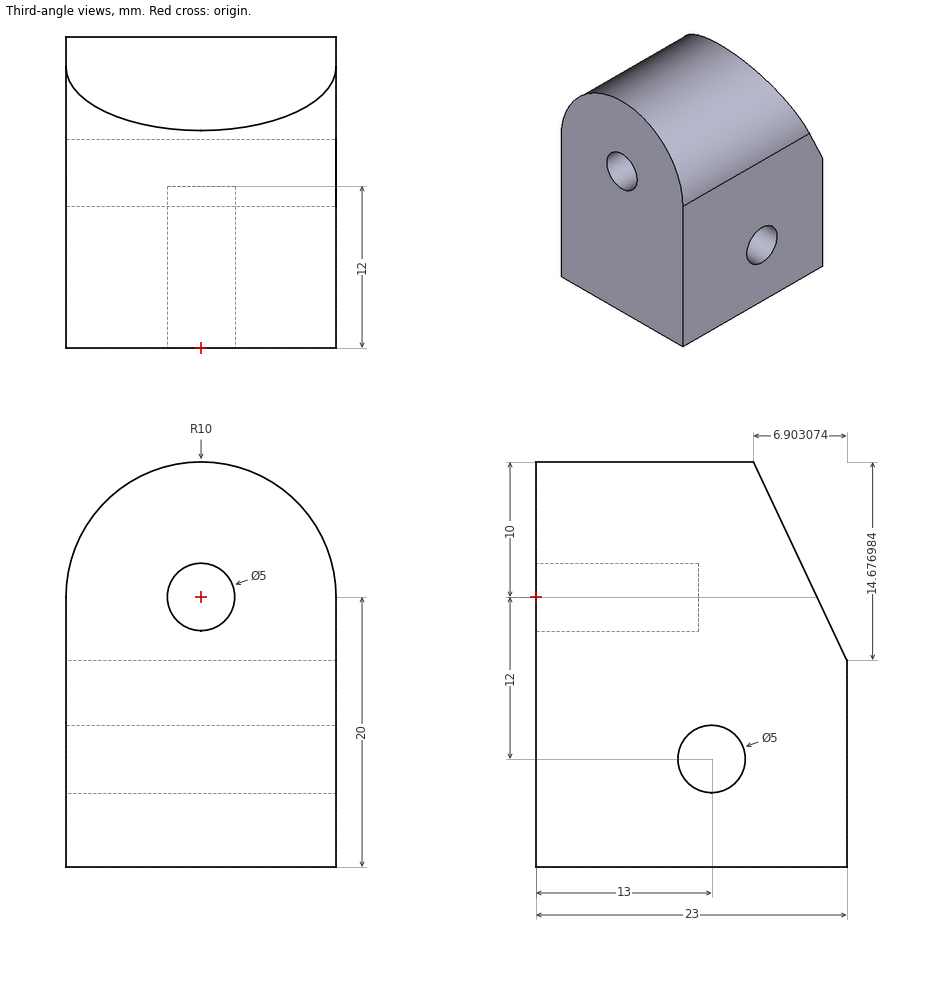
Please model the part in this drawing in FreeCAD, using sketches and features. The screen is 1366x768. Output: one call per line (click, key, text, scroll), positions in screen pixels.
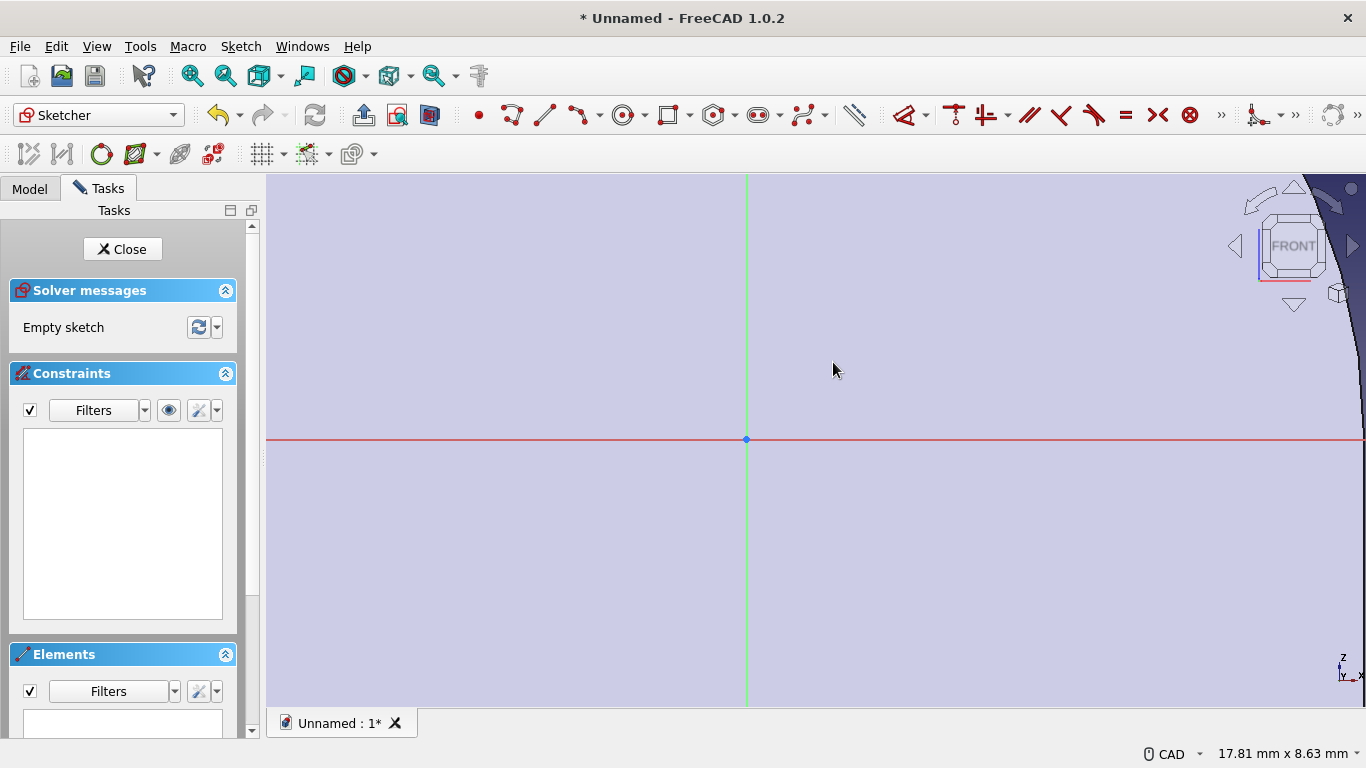
key(g)
key(c)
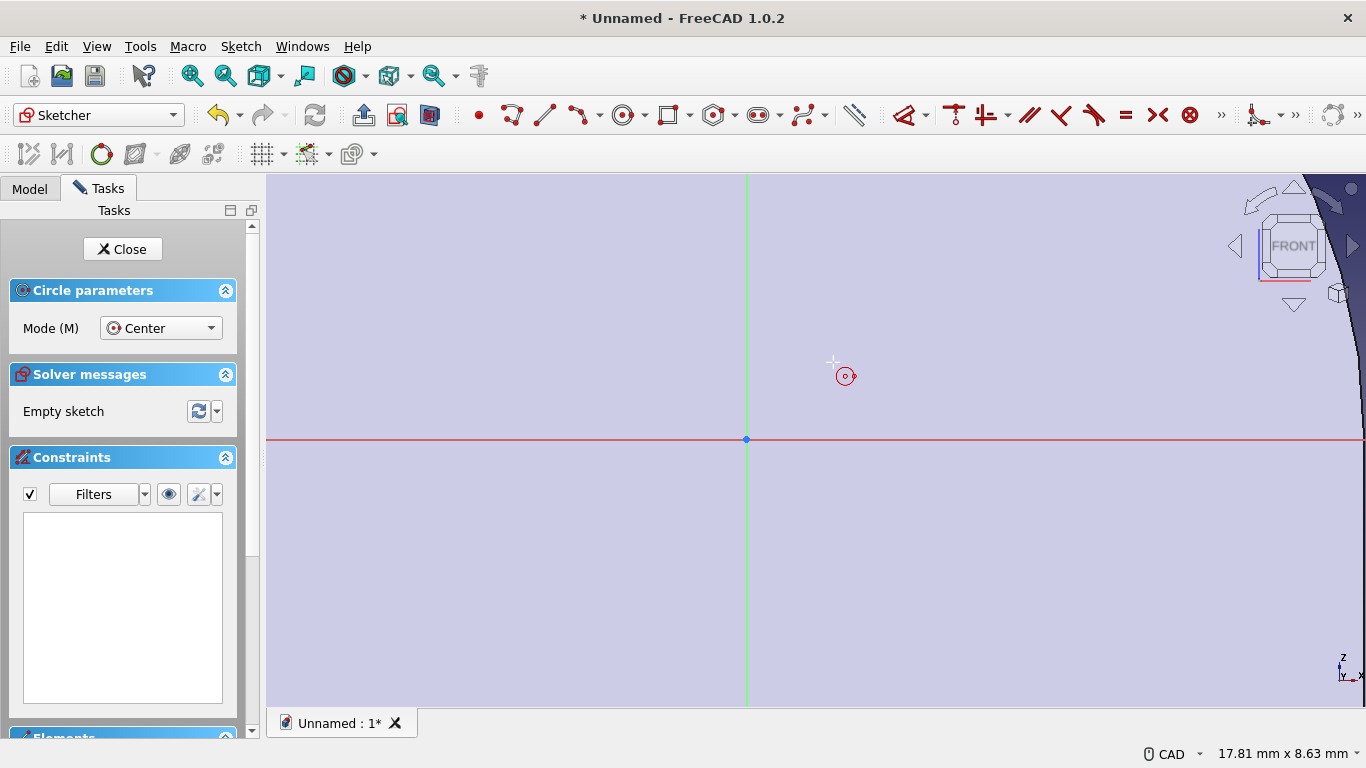
click(747, 440)
click(856, 331)
key(Escape)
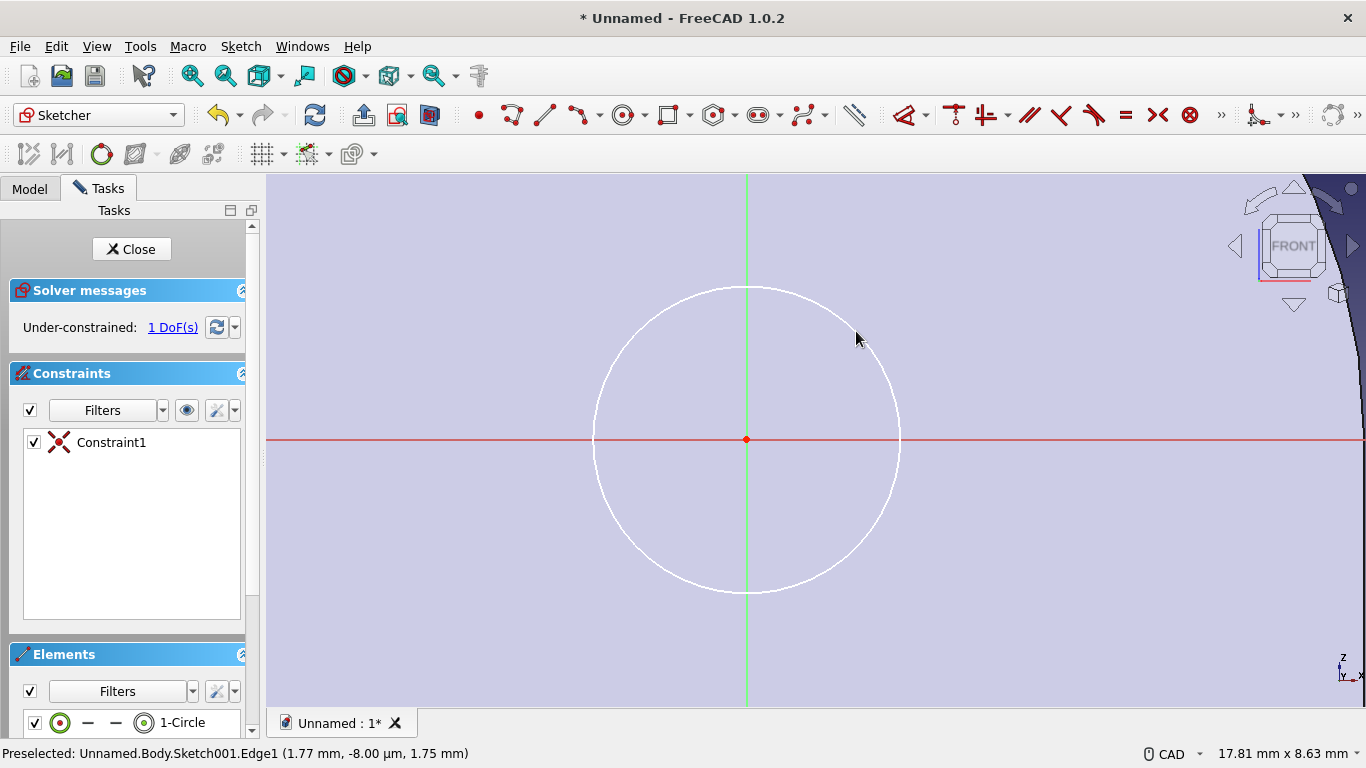
click(904, 116)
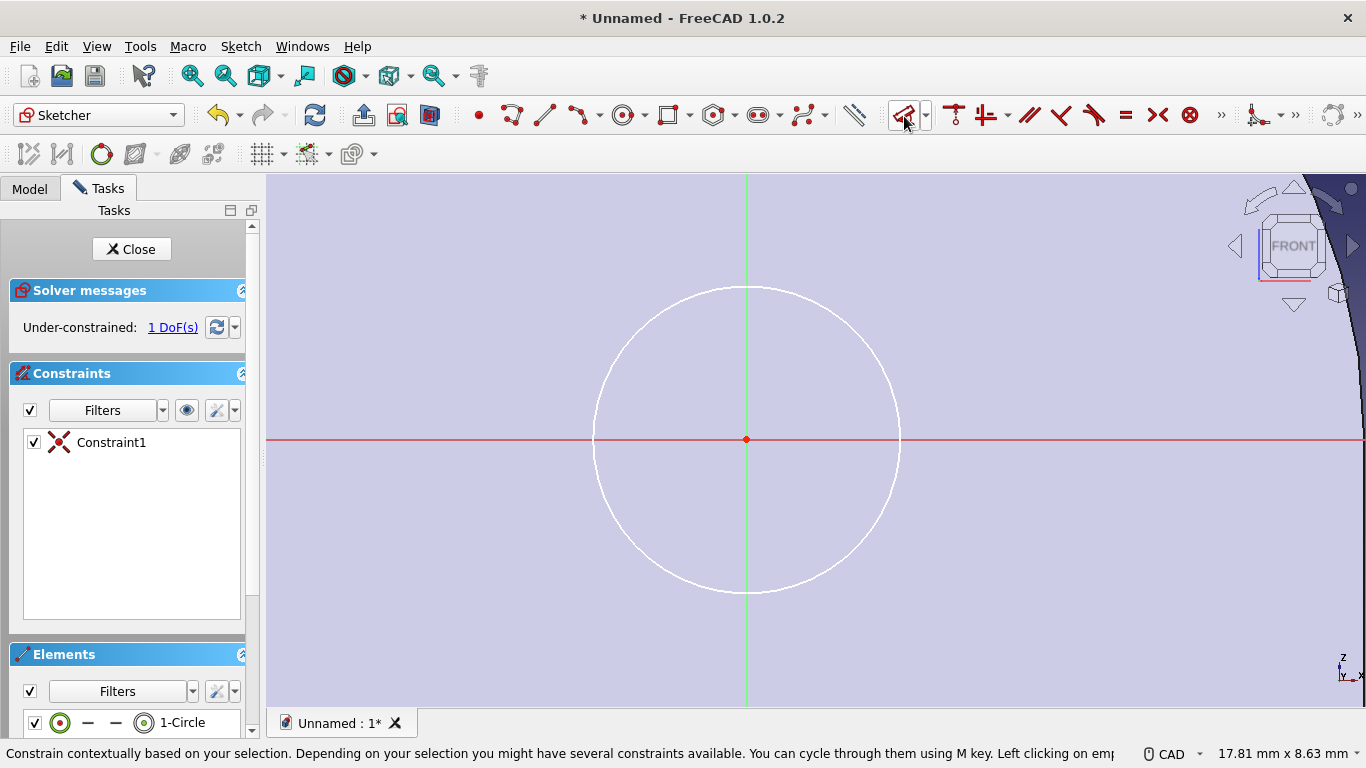
click(855, 331)
click(878, 308)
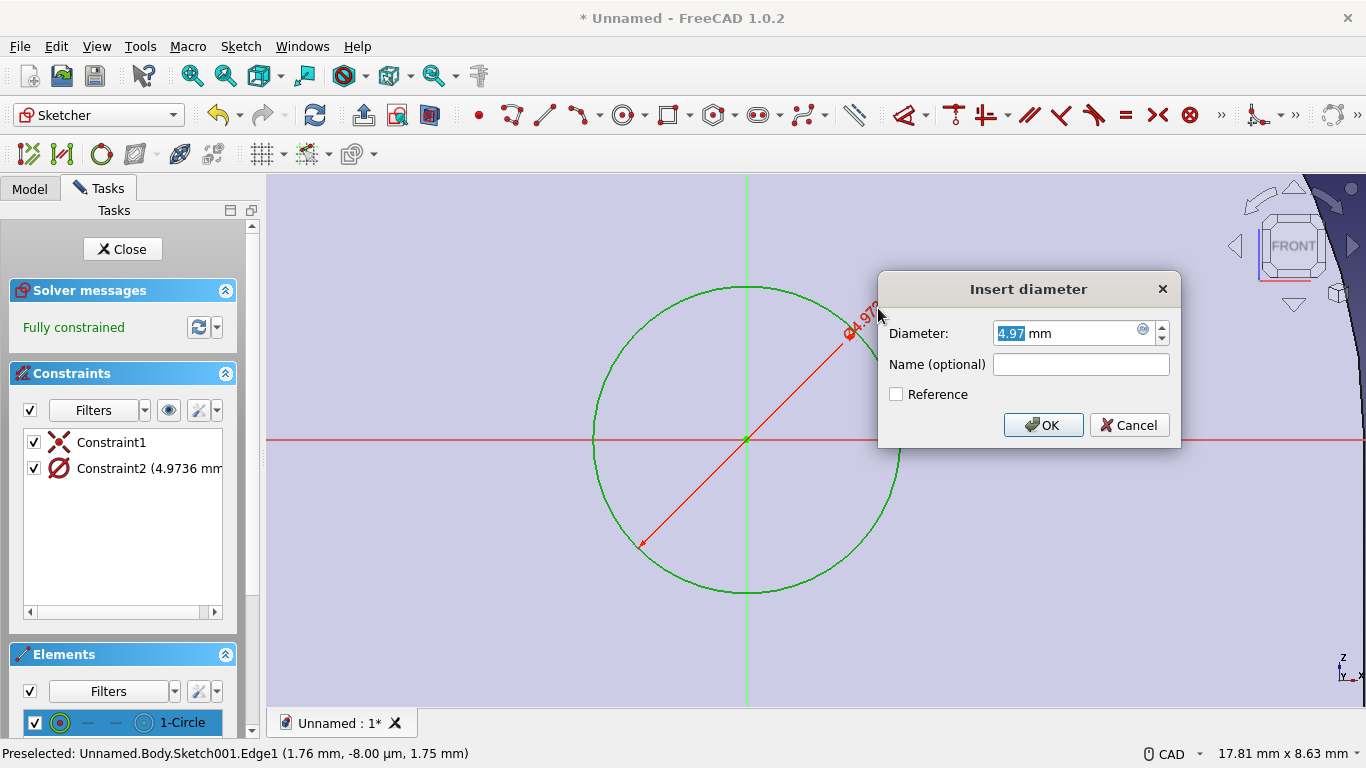
text(5)
key(Return)
key(Escape)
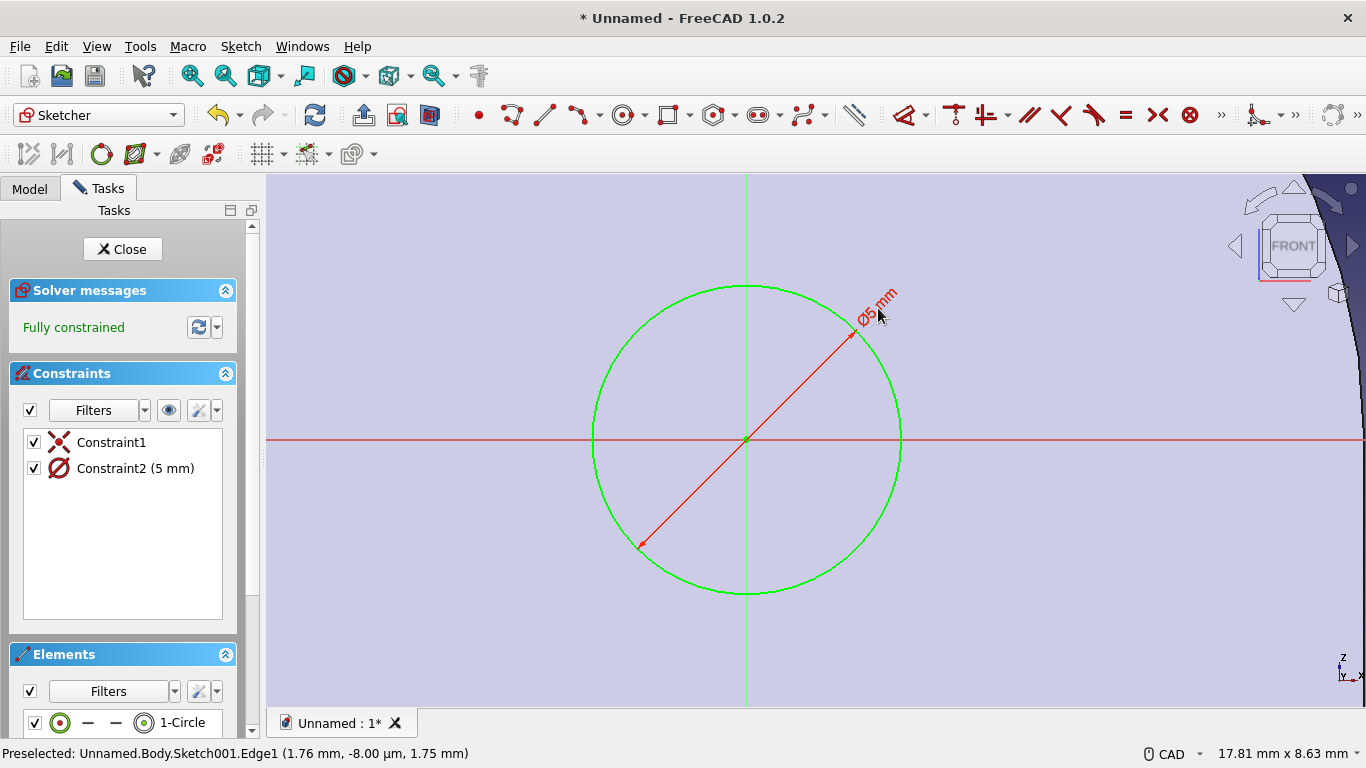
click(123, 249)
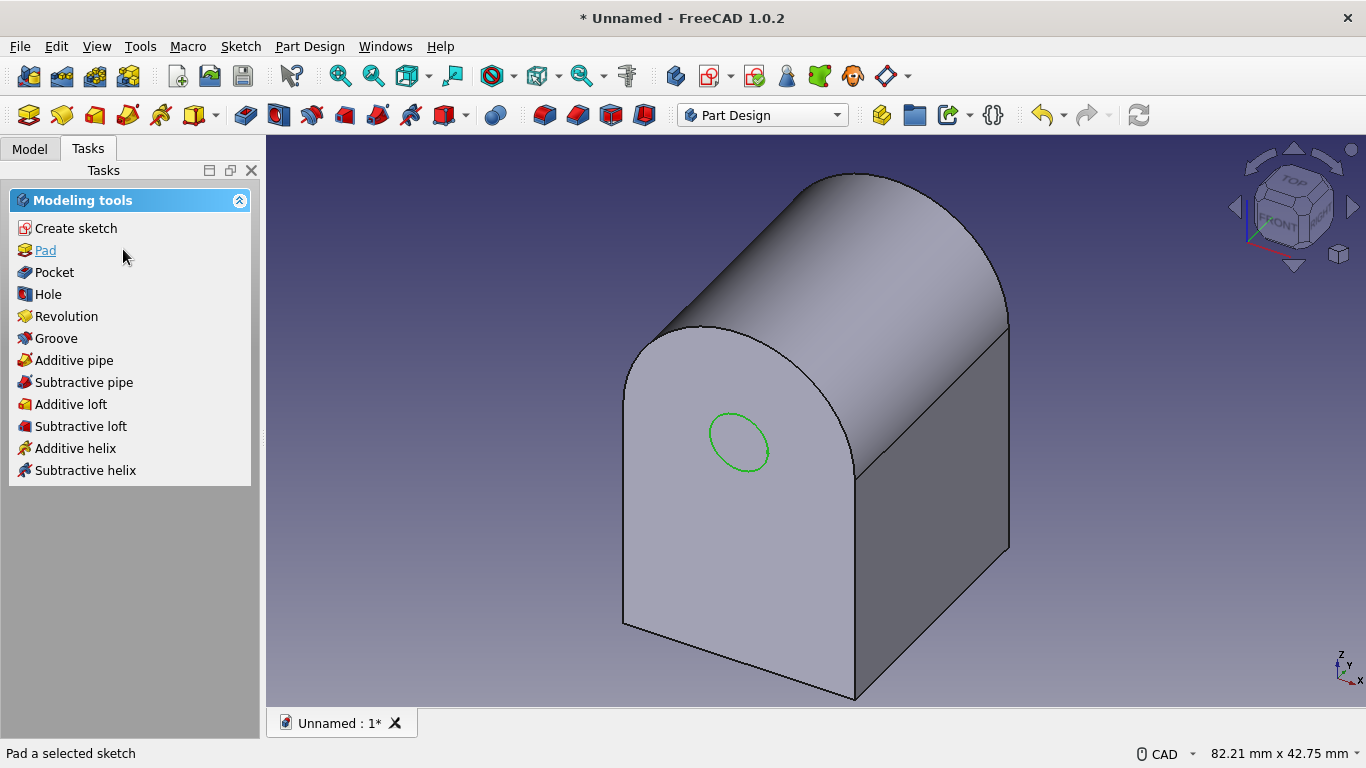
click(246, 116)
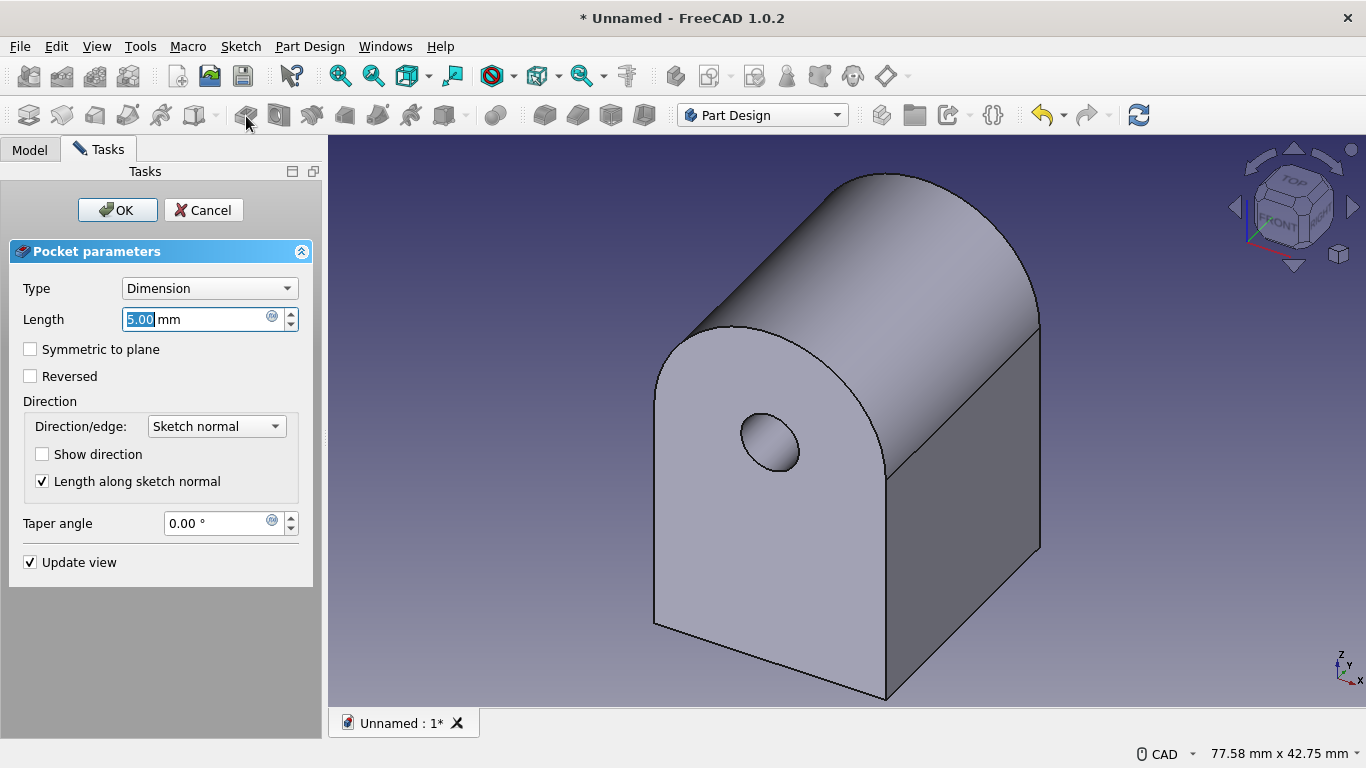
text(12)
key(Tab)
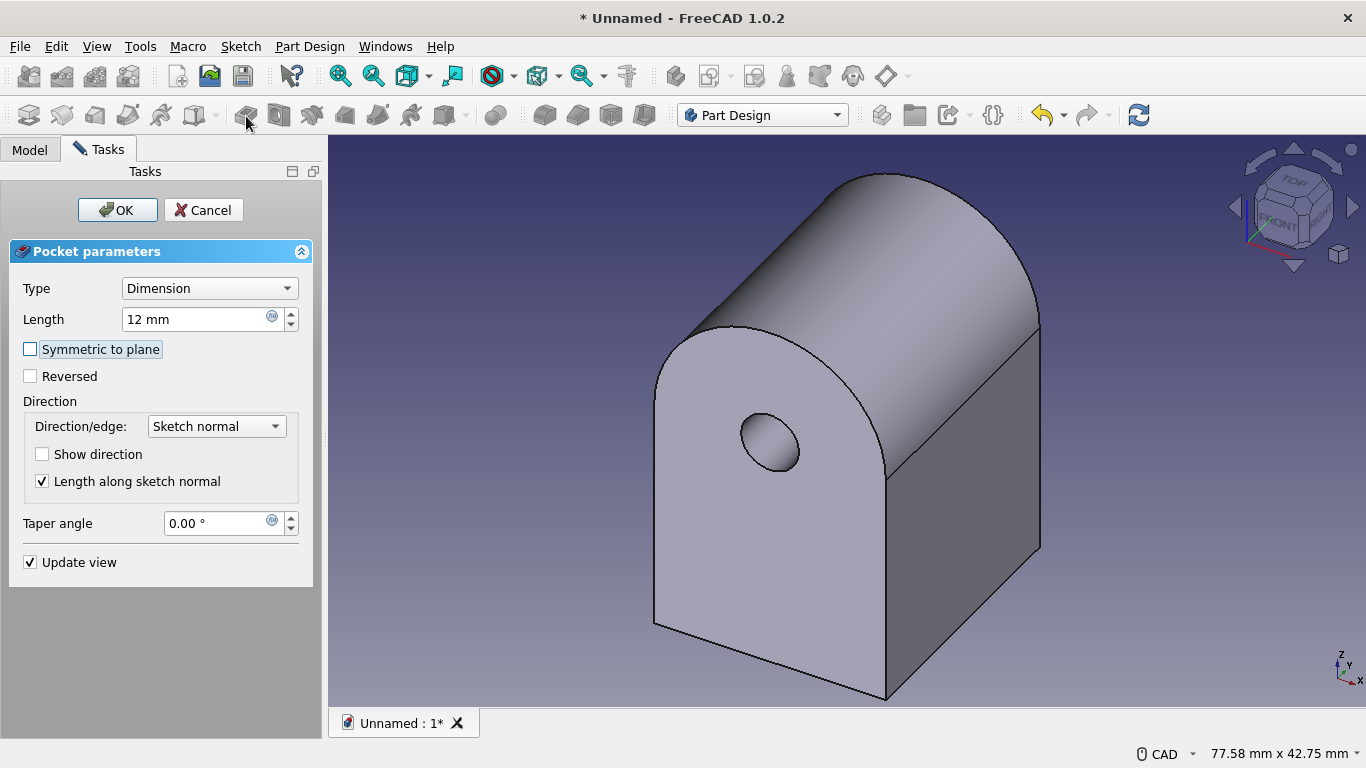
click(118, 210)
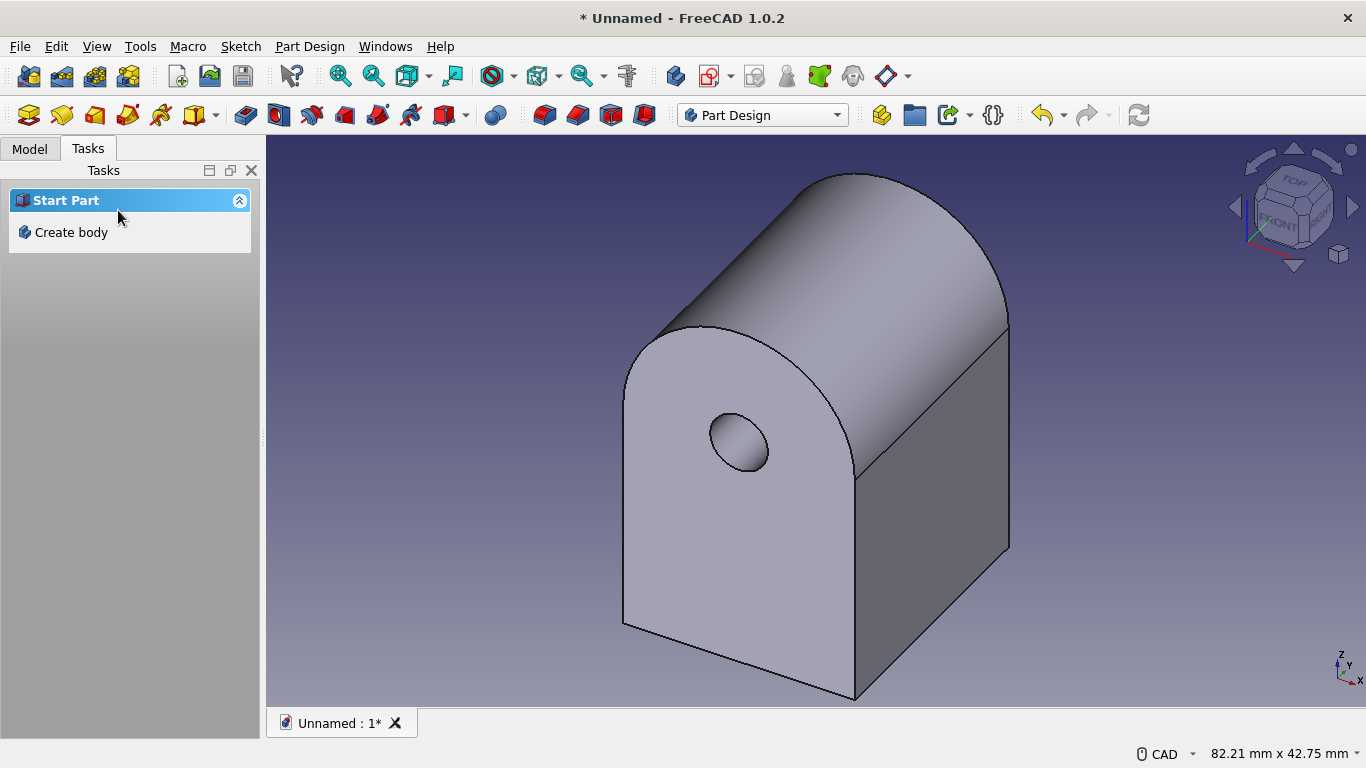
click(932, 513)